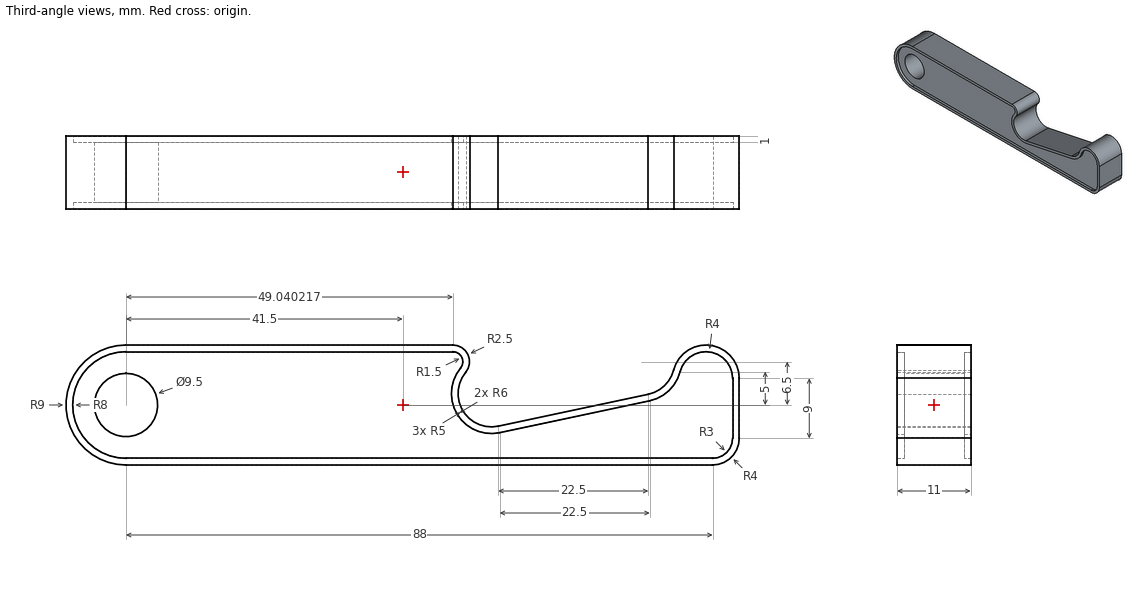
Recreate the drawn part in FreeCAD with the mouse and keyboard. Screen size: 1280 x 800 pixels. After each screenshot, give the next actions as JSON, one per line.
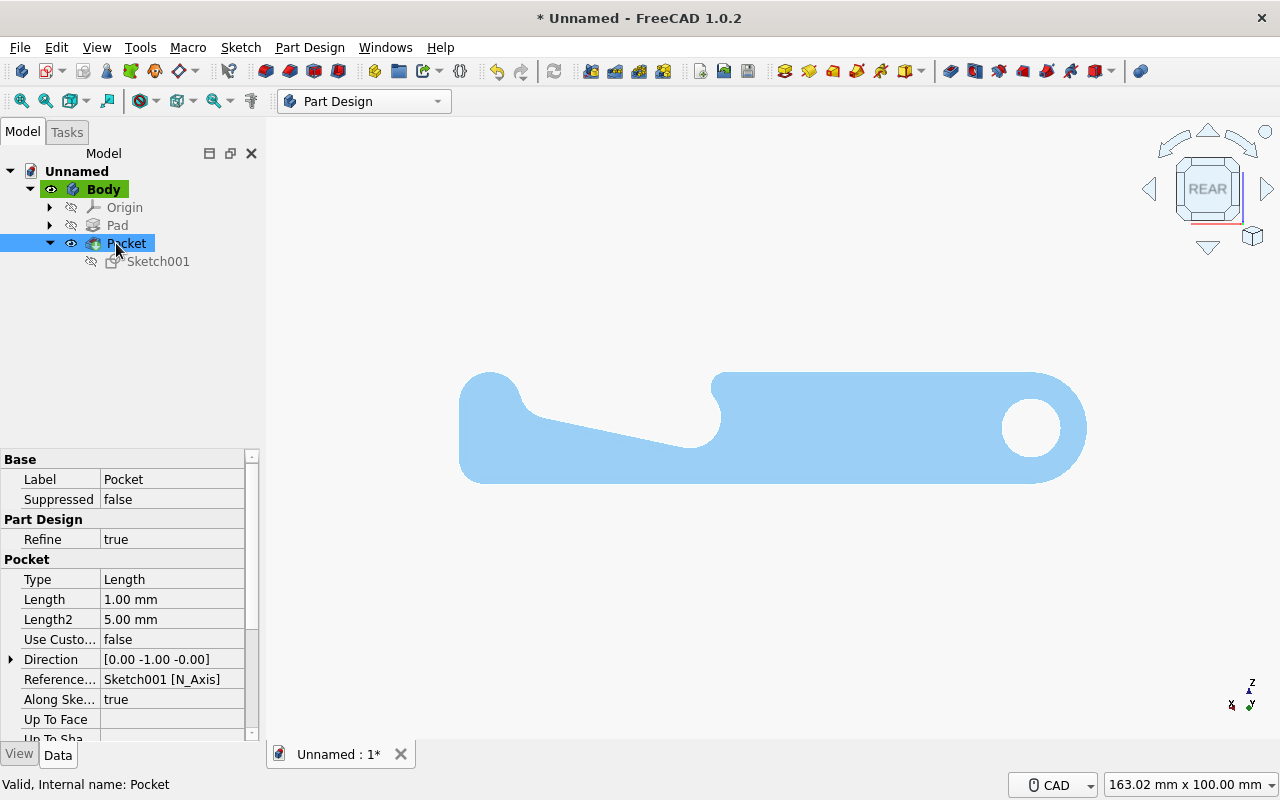
{"action": "left_click", "coordinate": [592, 72]}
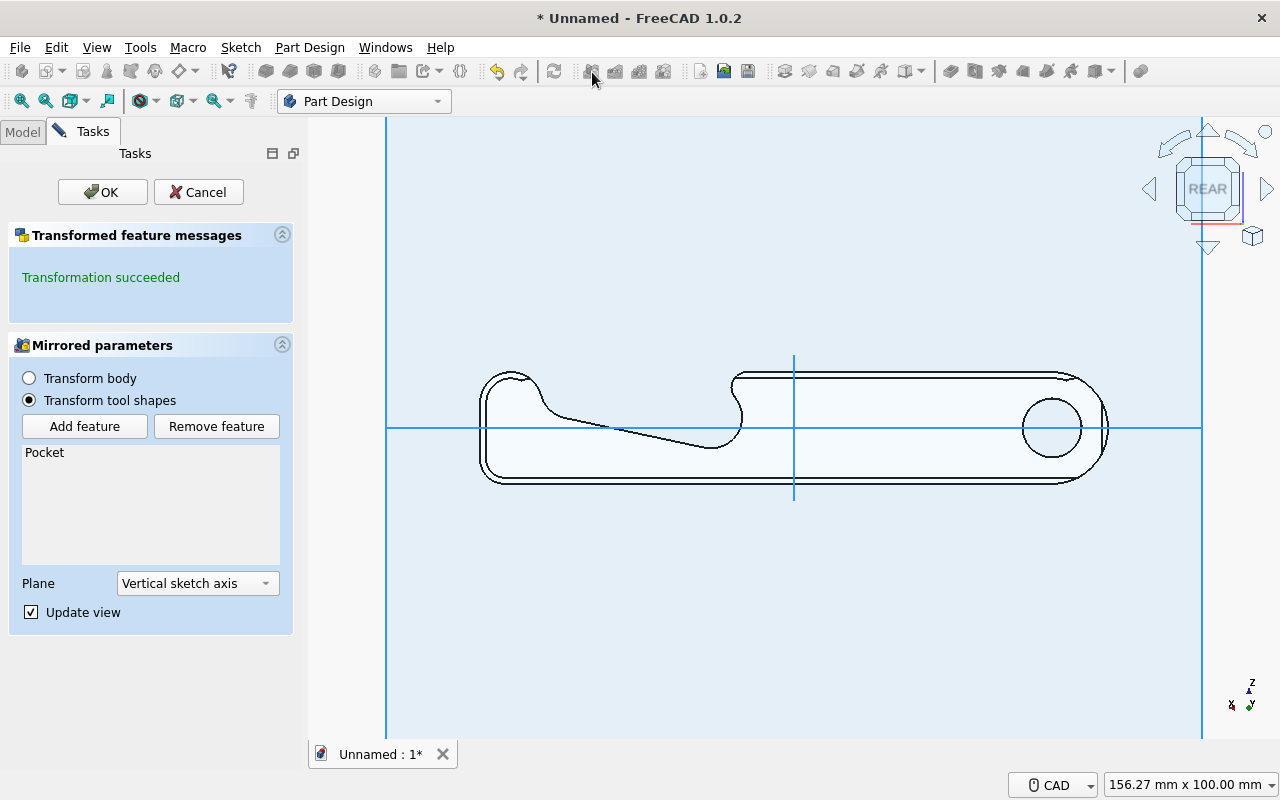
{"action": "left_click", "coordinate": [198, 584]}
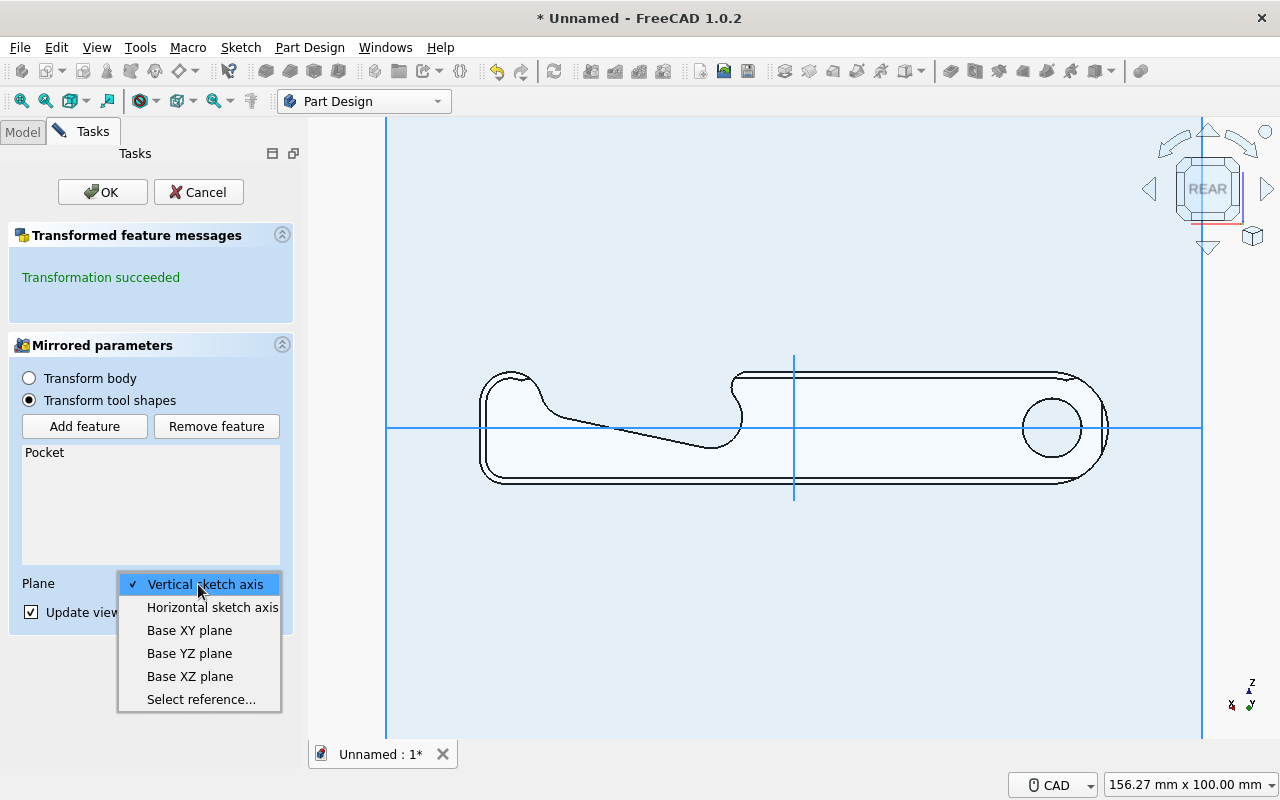
{"action": "left_click", "coordinate": [198, 676]}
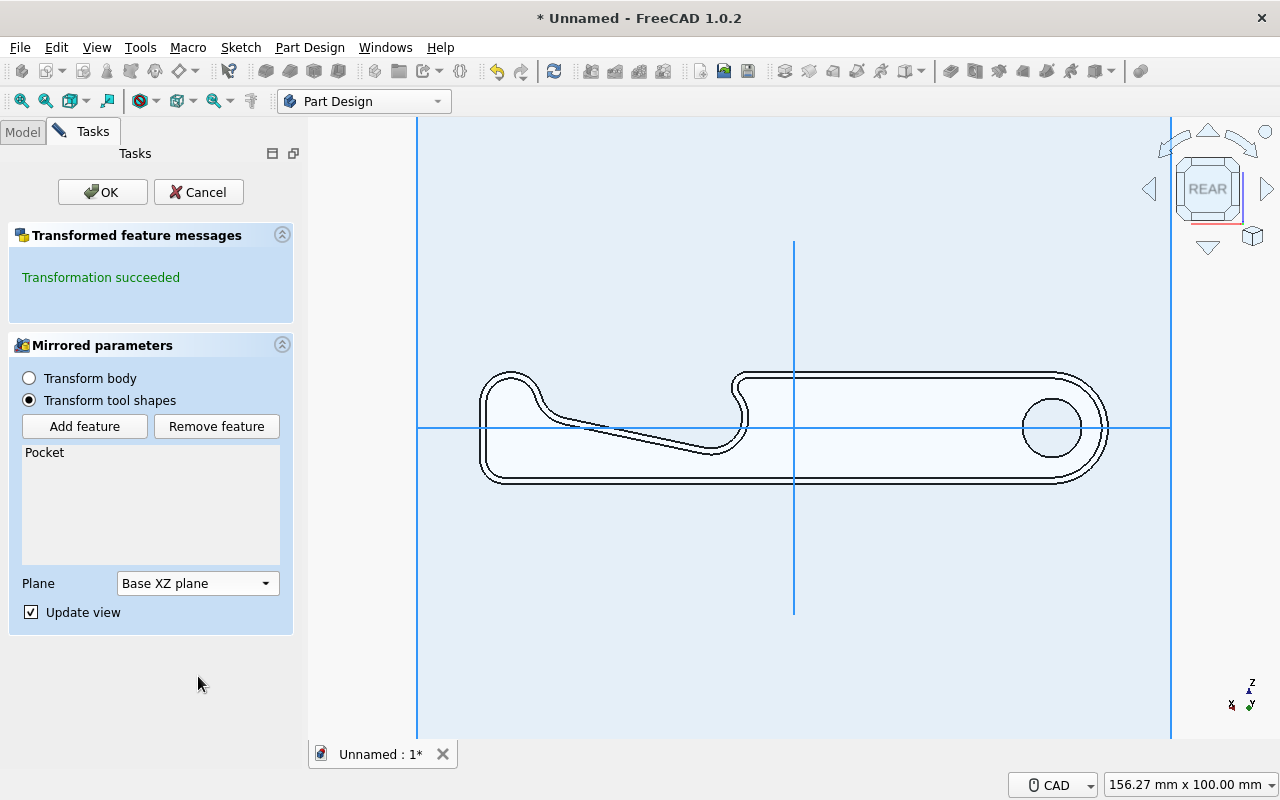
{"action": "left_click", "coordinate": [103, 192]}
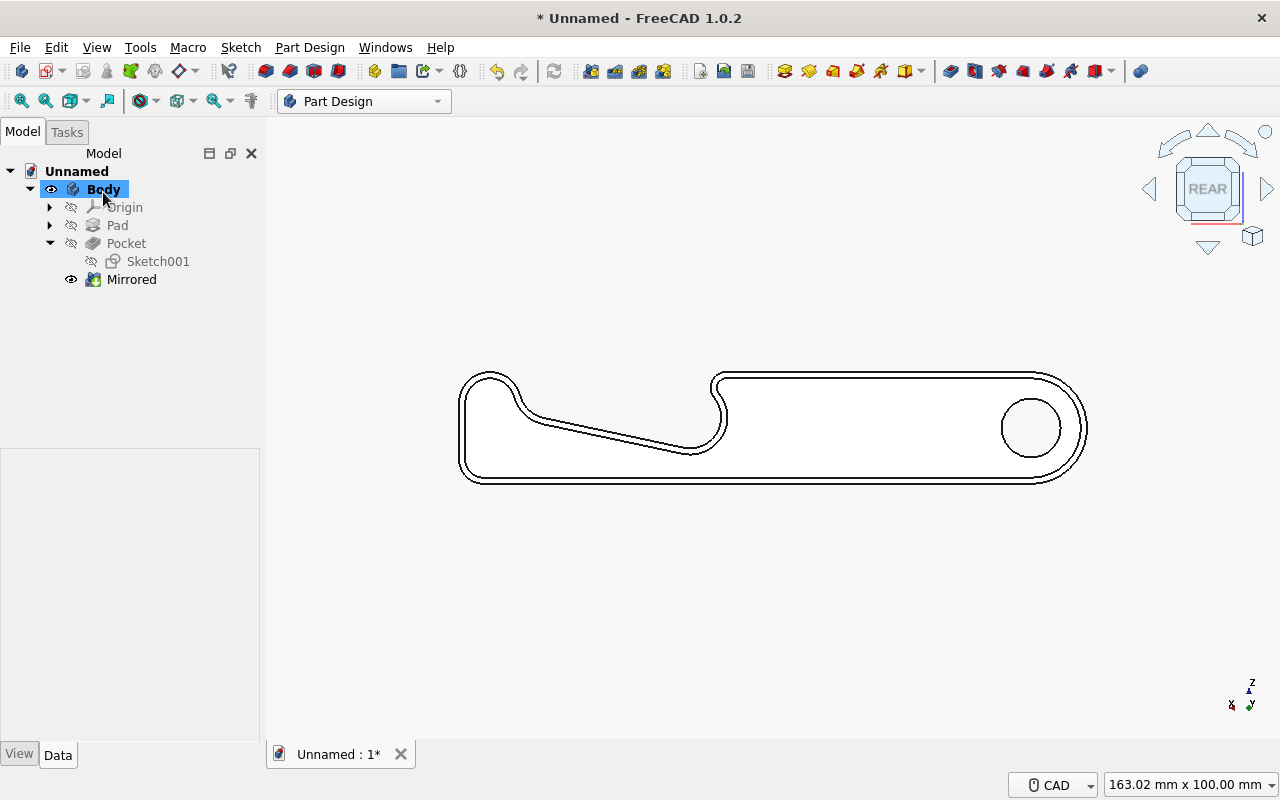
{"action": "key", "text": "0"}